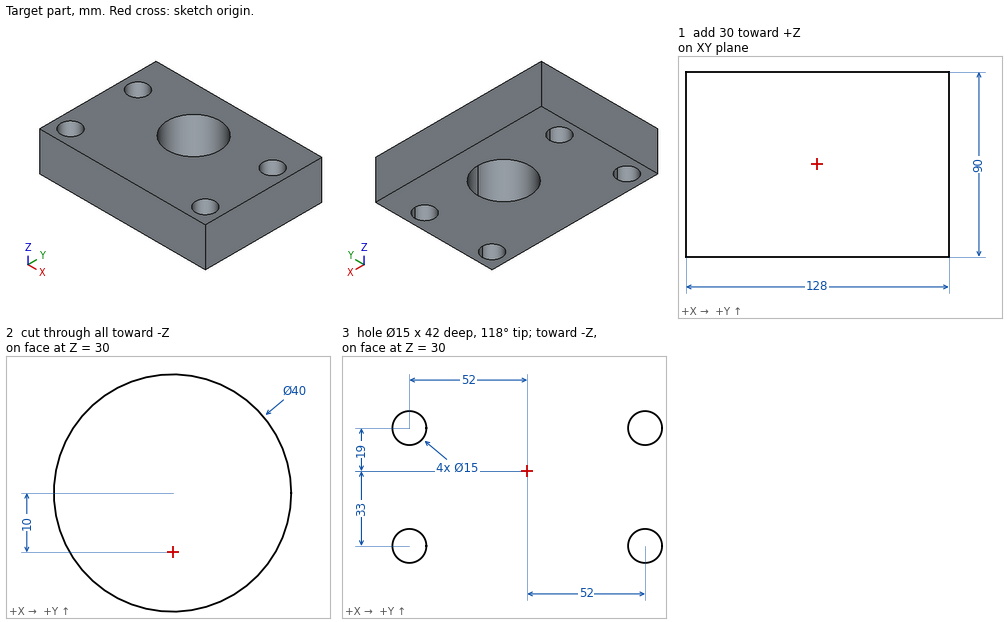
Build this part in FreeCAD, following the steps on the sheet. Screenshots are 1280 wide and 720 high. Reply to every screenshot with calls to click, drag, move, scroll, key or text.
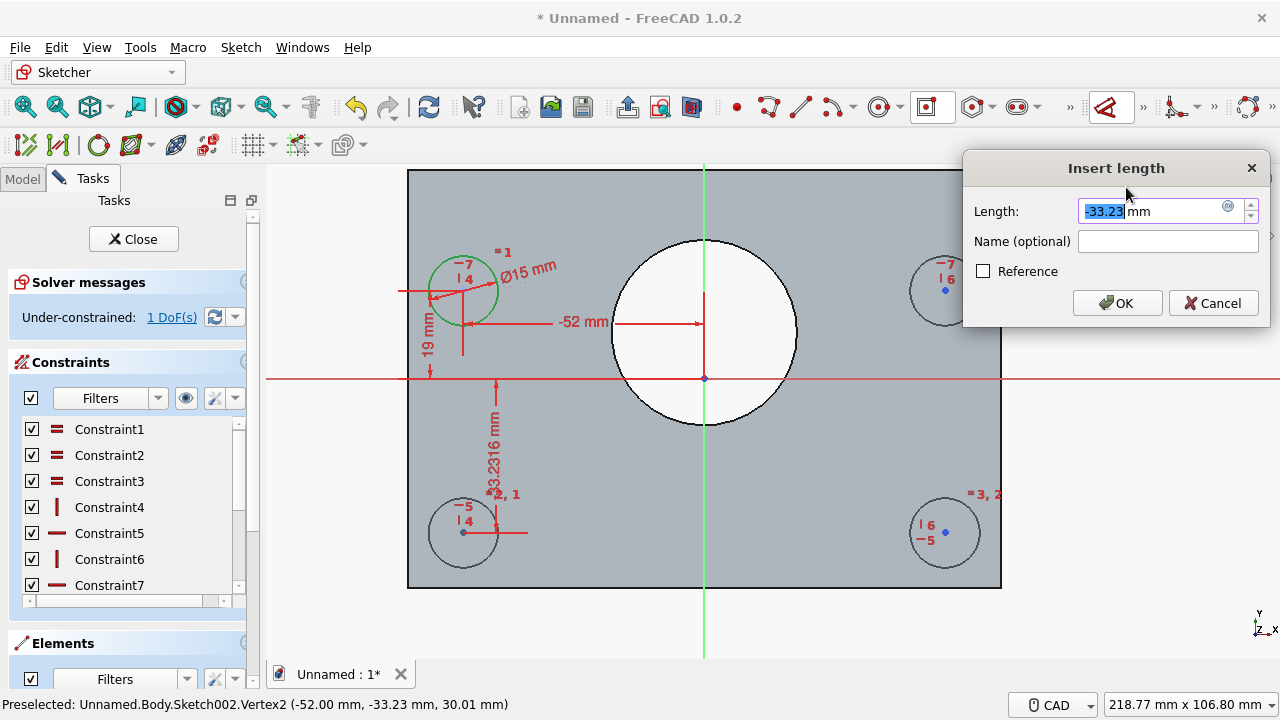
text(-33)
key(Return)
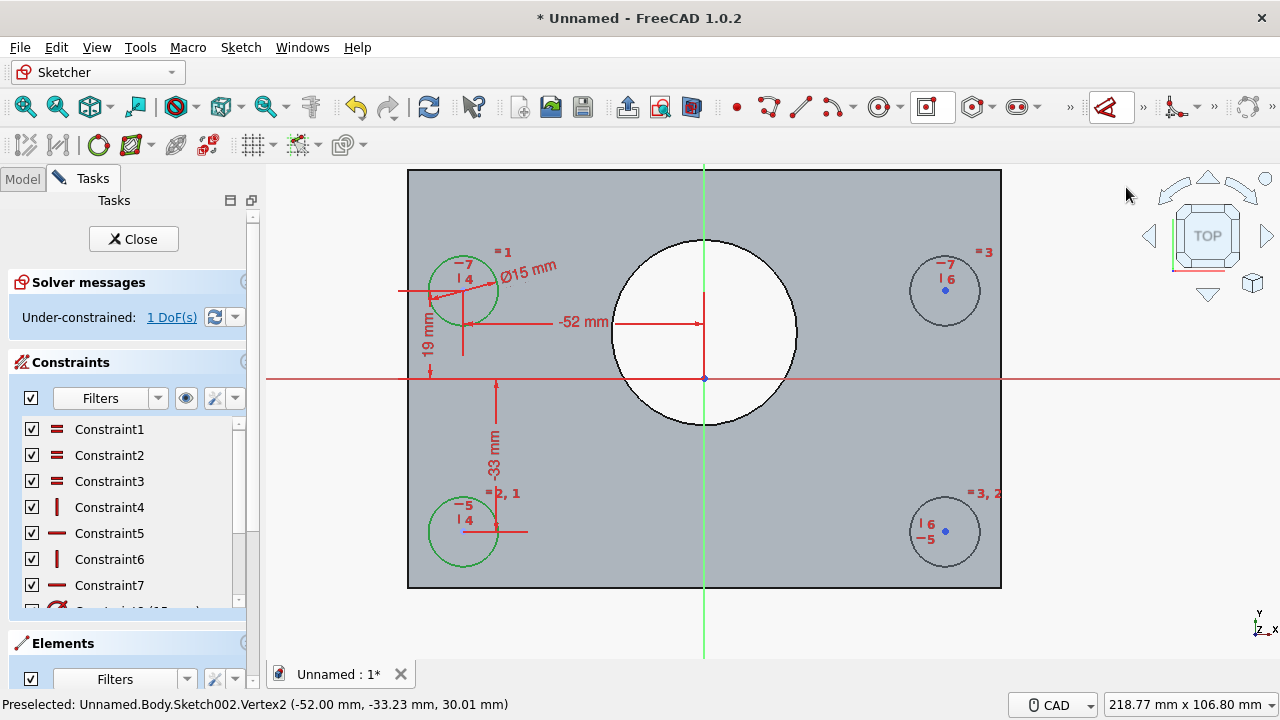
click(945, 532)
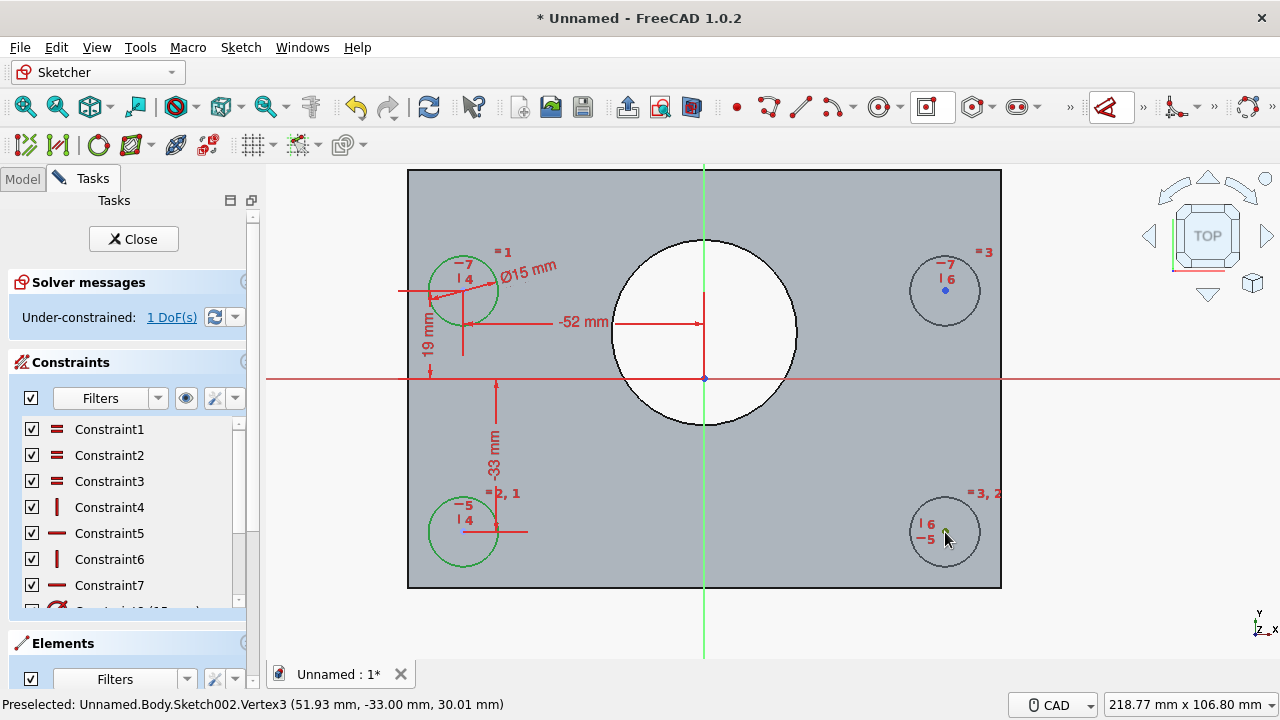
click(1128, 108)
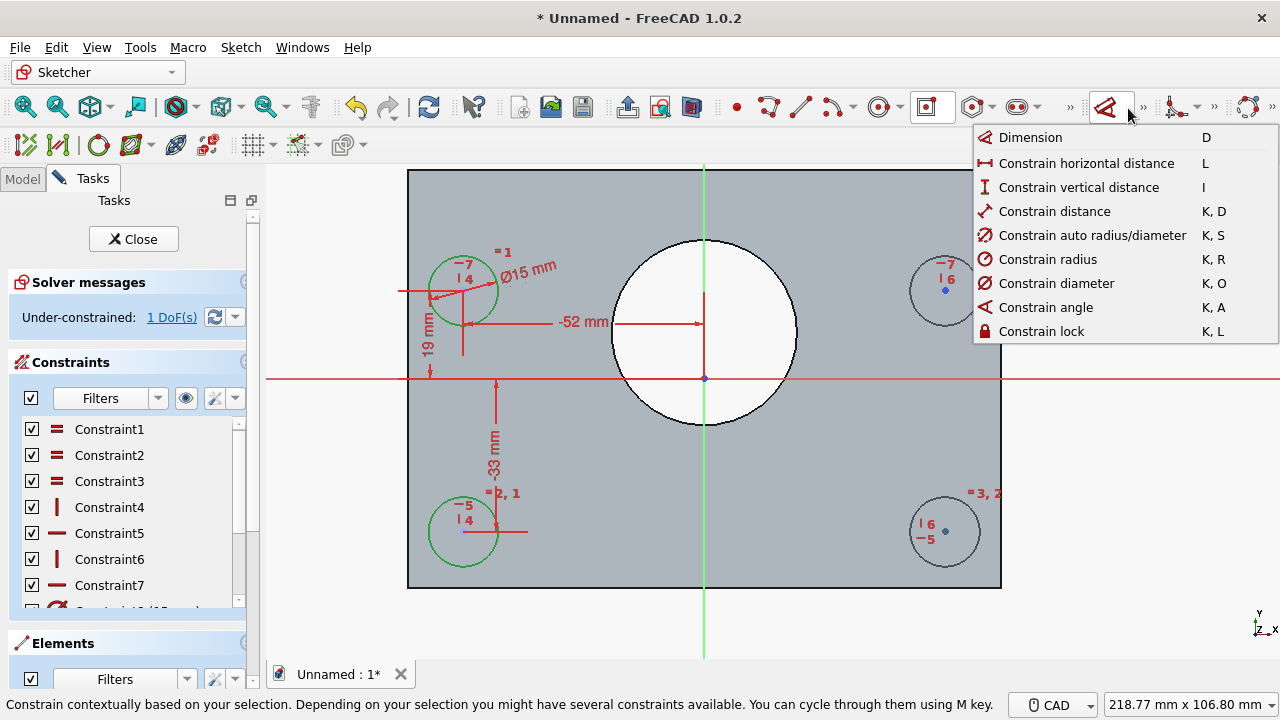
click(1126, 163)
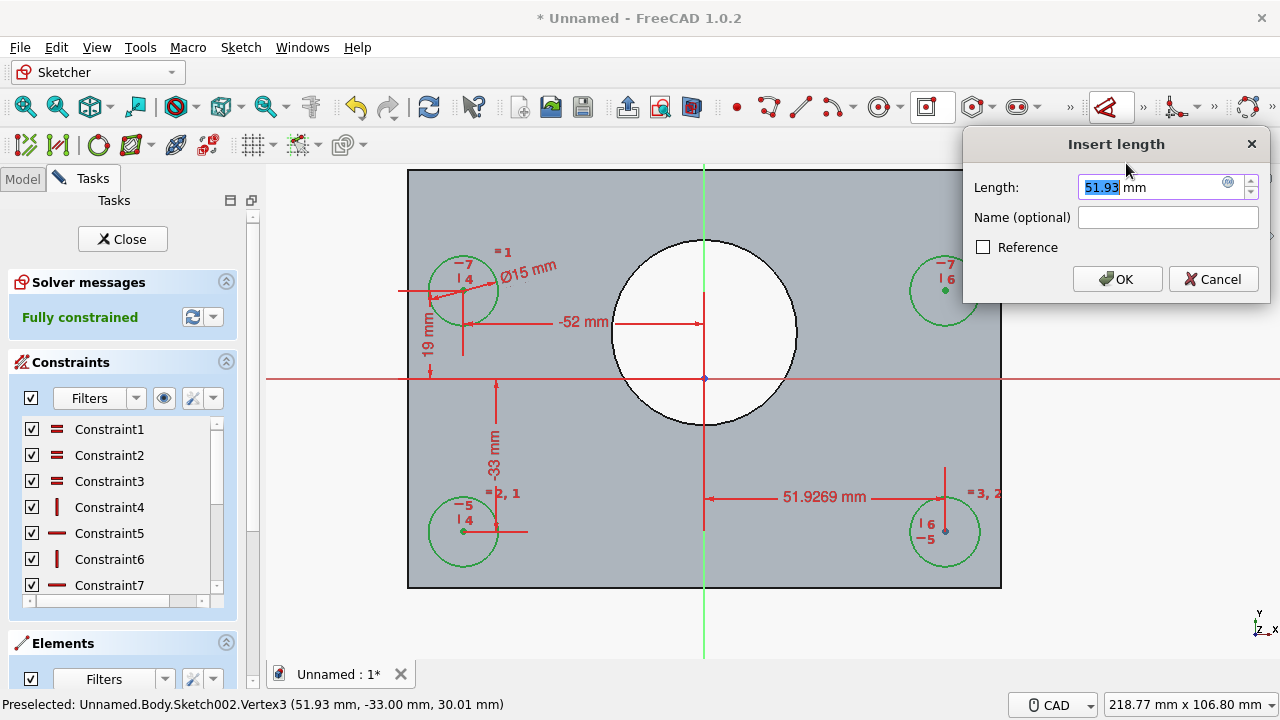
text(52)
key(Return)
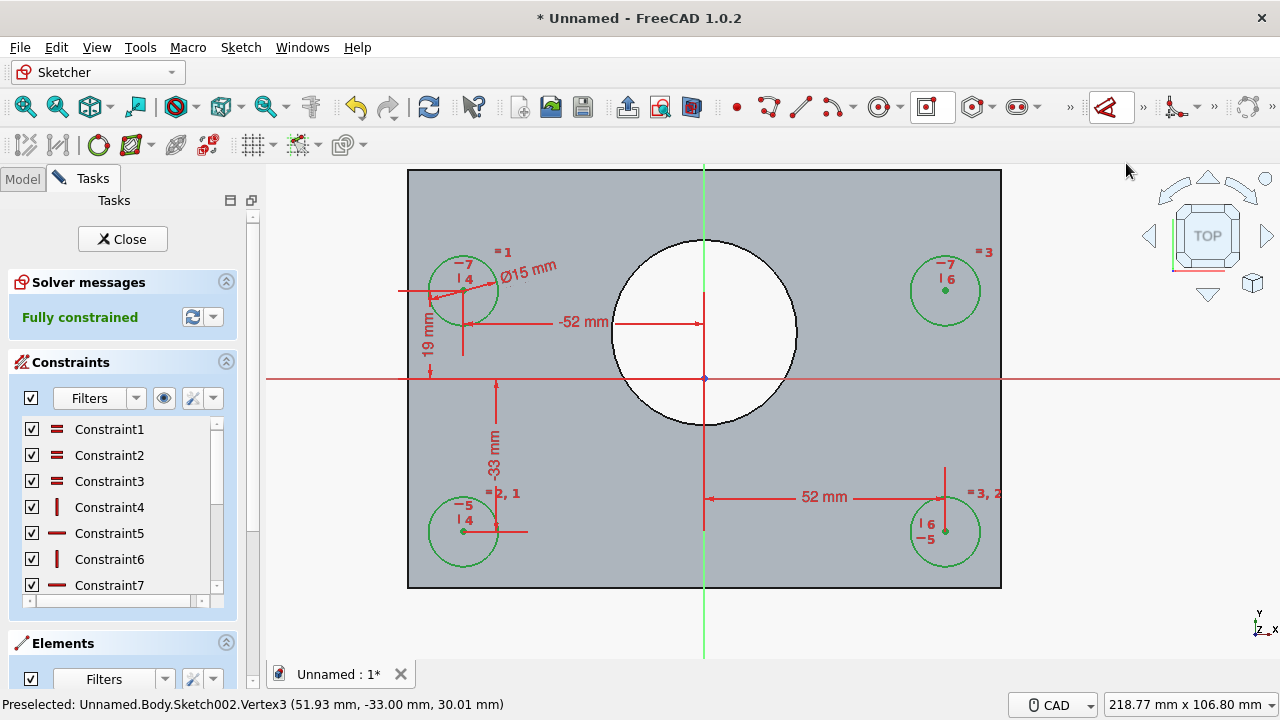
click(123, 239)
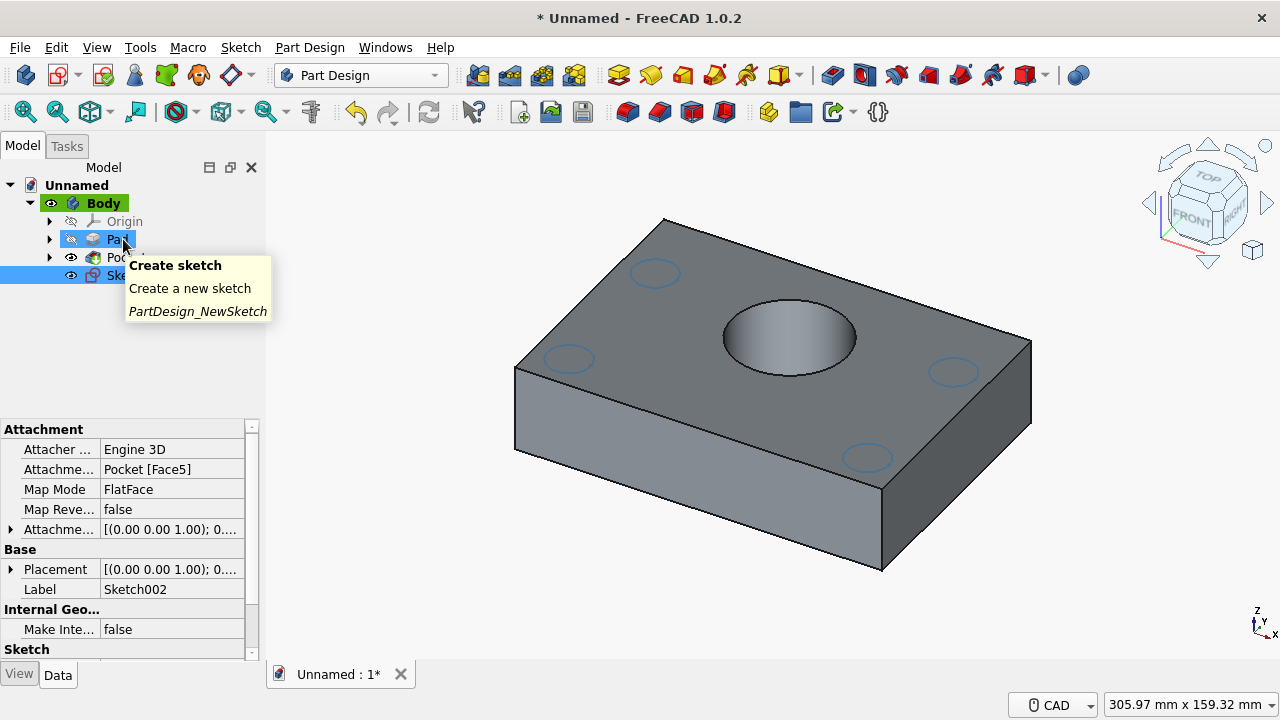
click(866, 76)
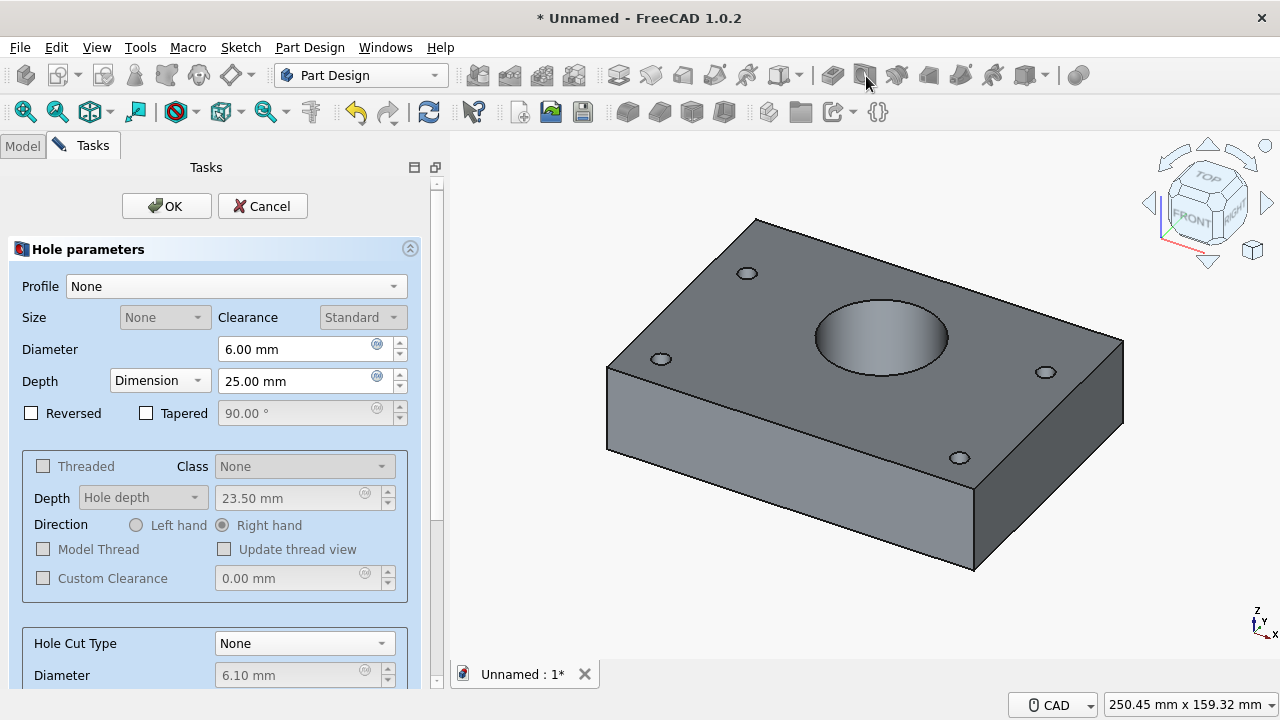
triple_click(305, 349)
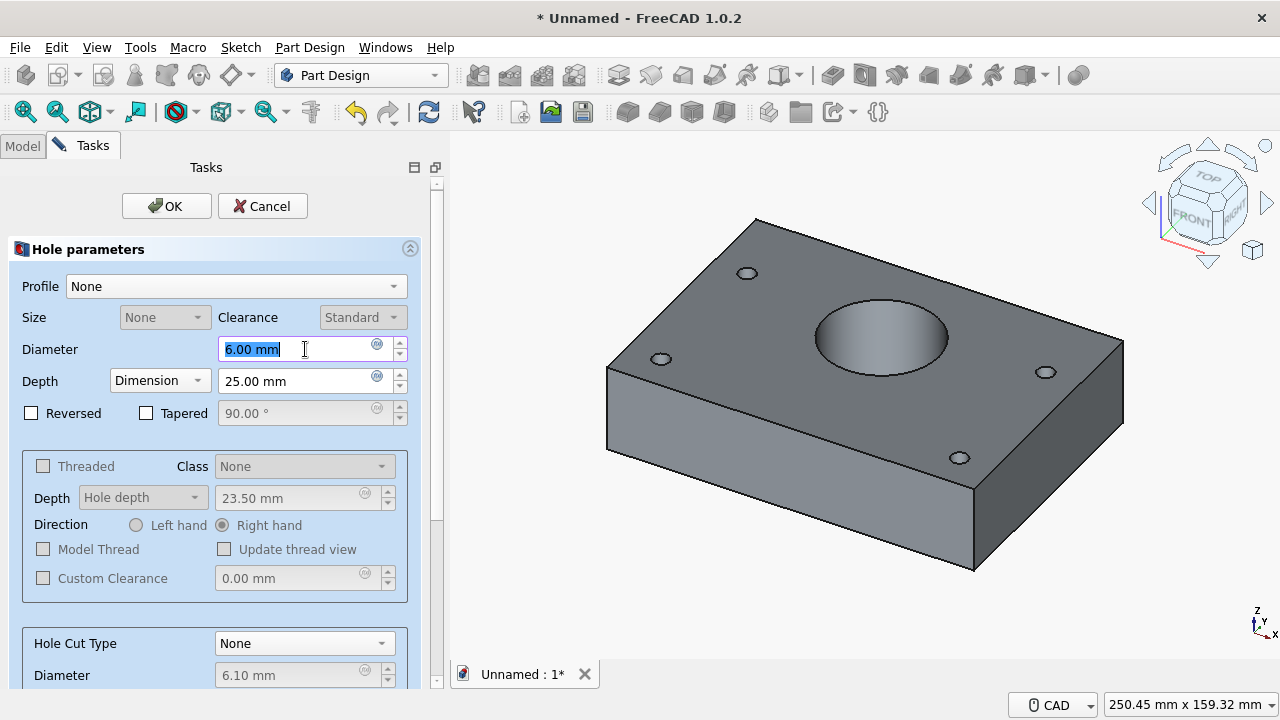
text(15)
key(Tab)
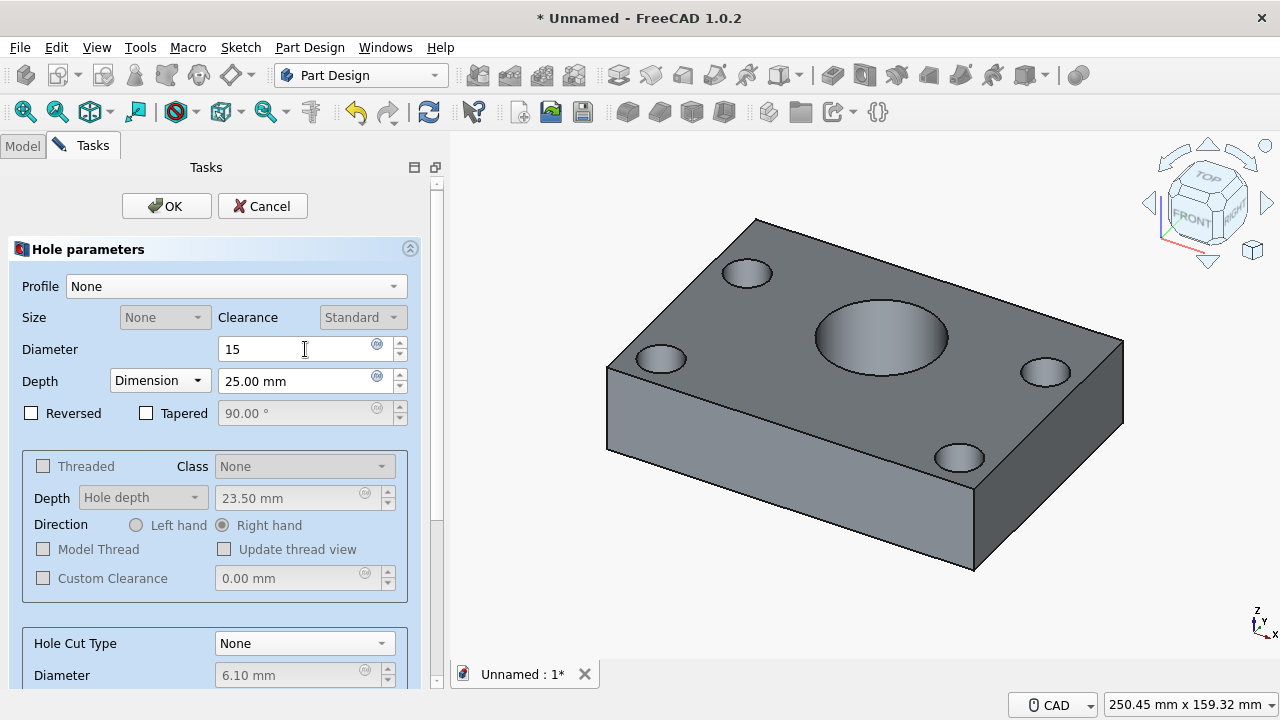
triple_click(305, 381)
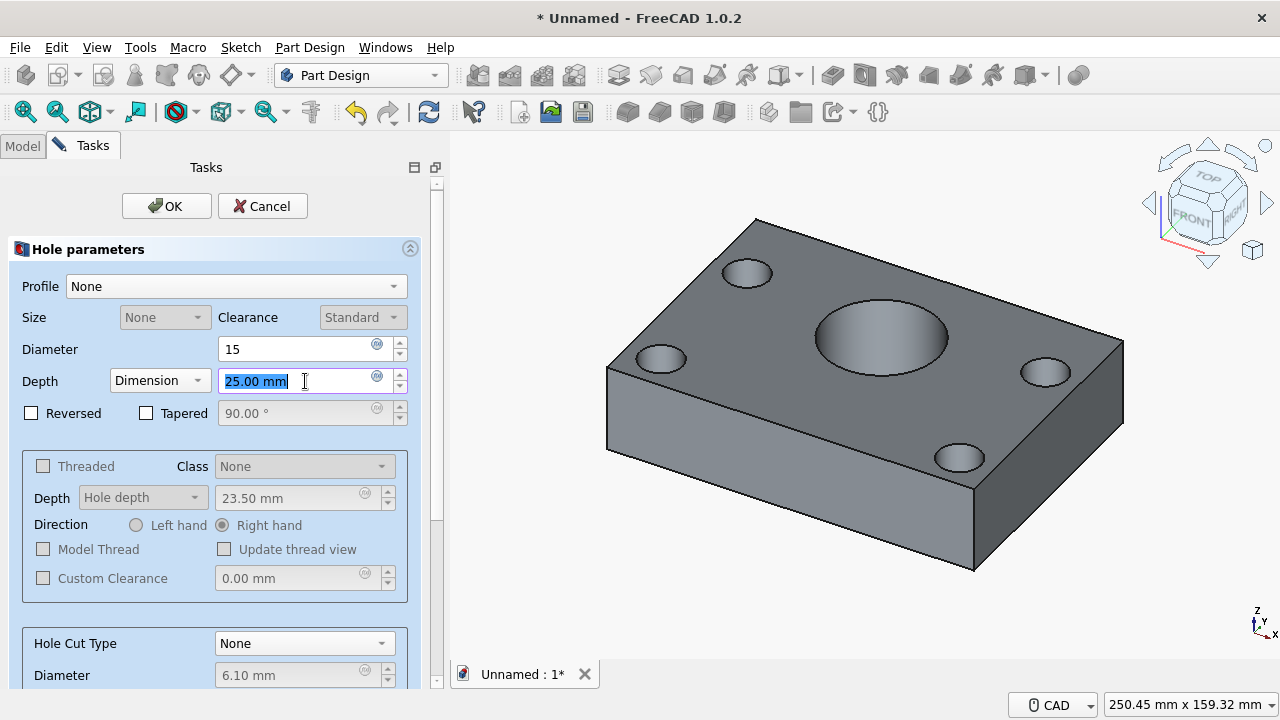
text(42)
key(Tab)